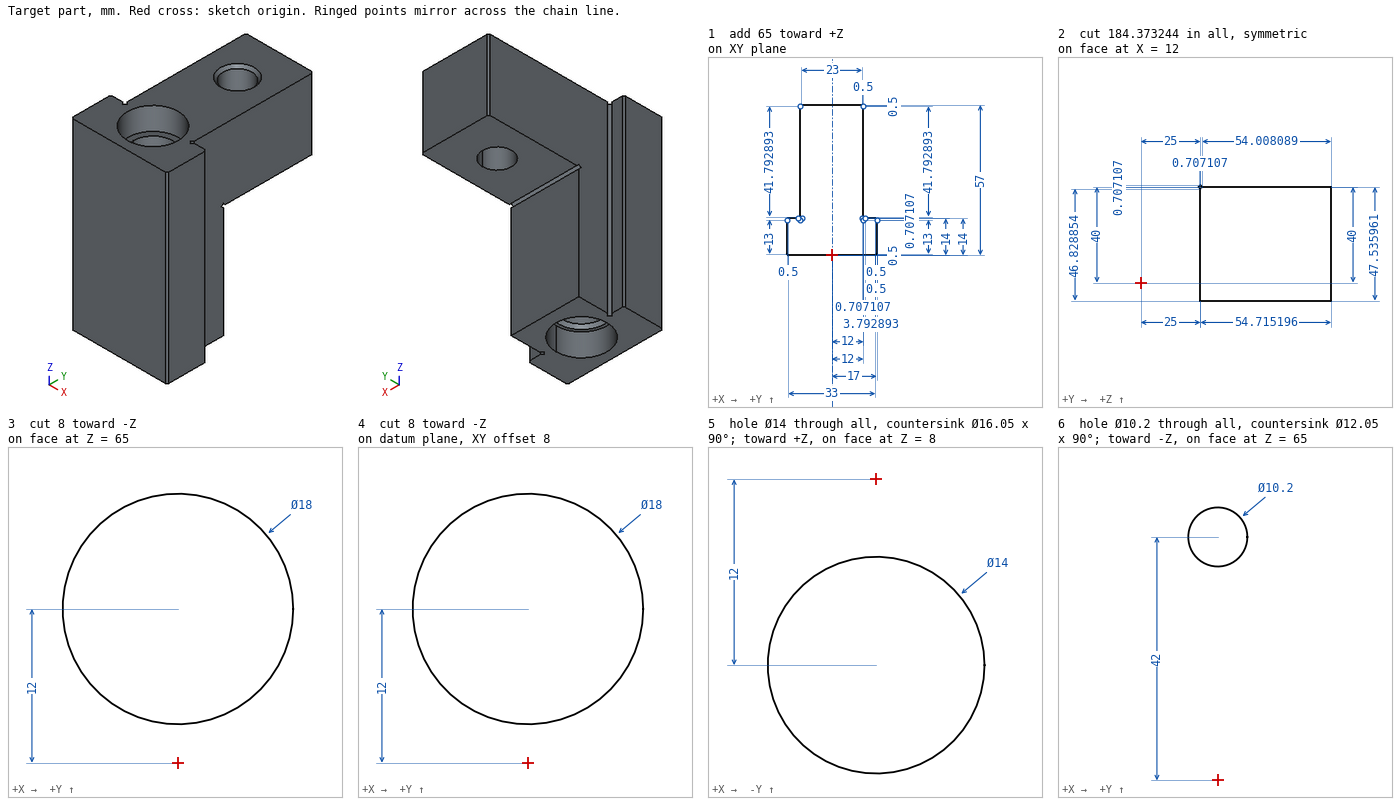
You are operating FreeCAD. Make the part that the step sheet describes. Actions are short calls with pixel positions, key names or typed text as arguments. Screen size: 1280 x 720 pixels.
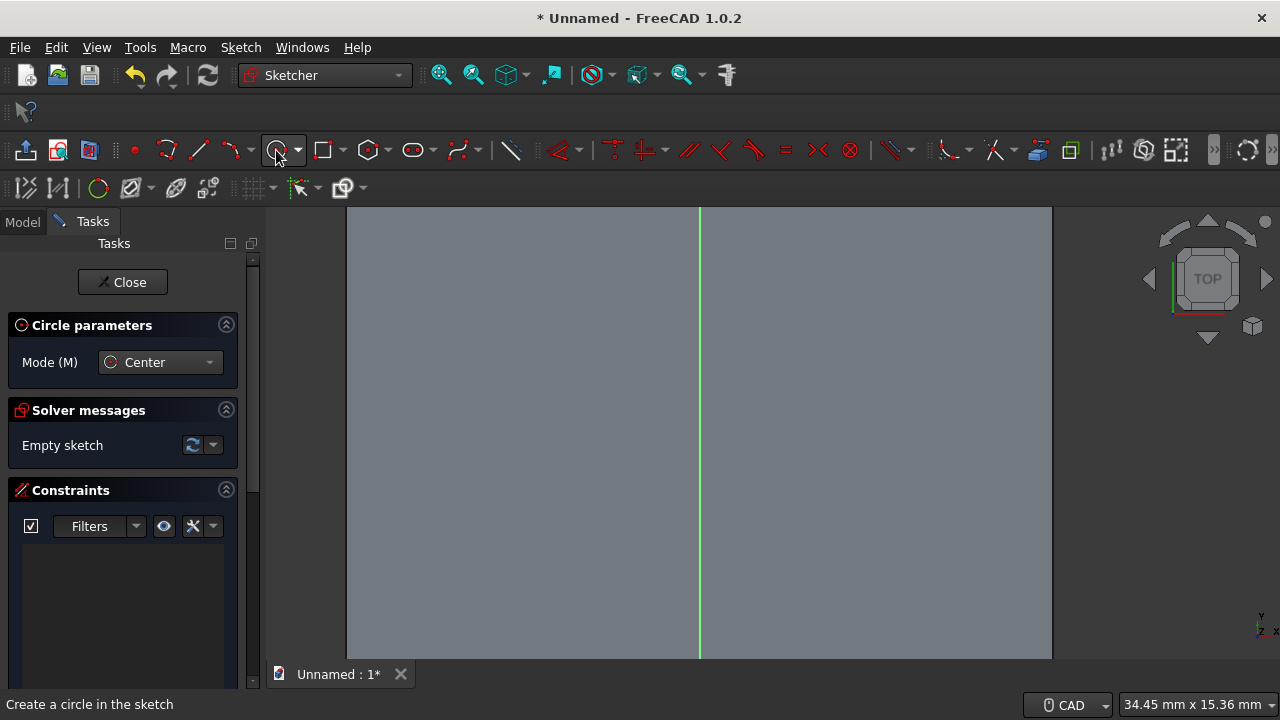
click(700, 433)
click(806, 327)
key(Escape)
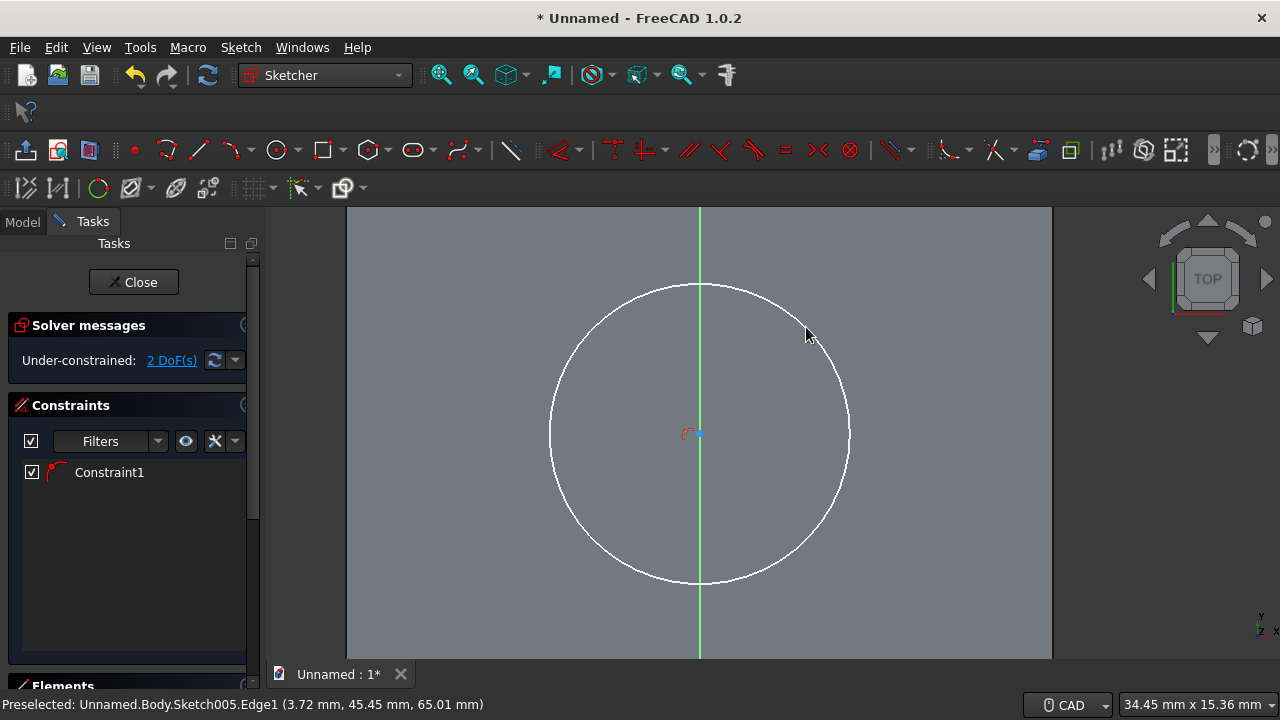
key(d)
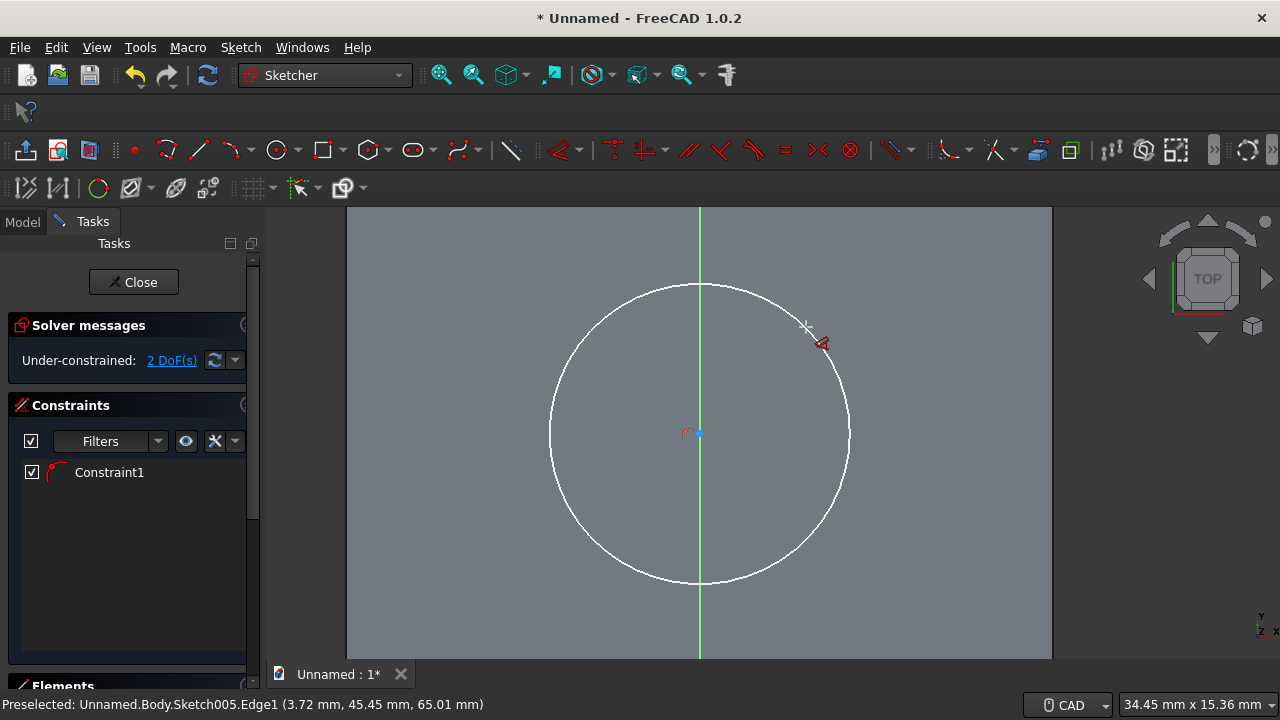
click(806, 328)
click(829, 305)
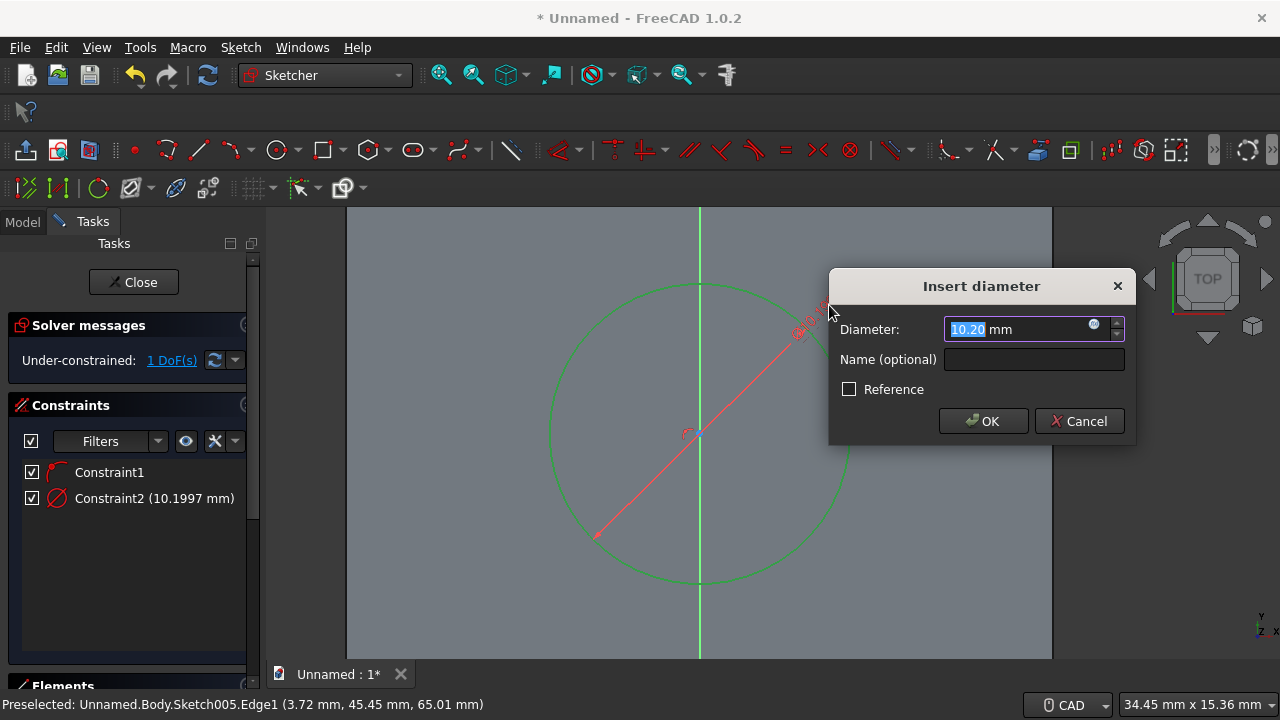
text(10.2)
key(Return)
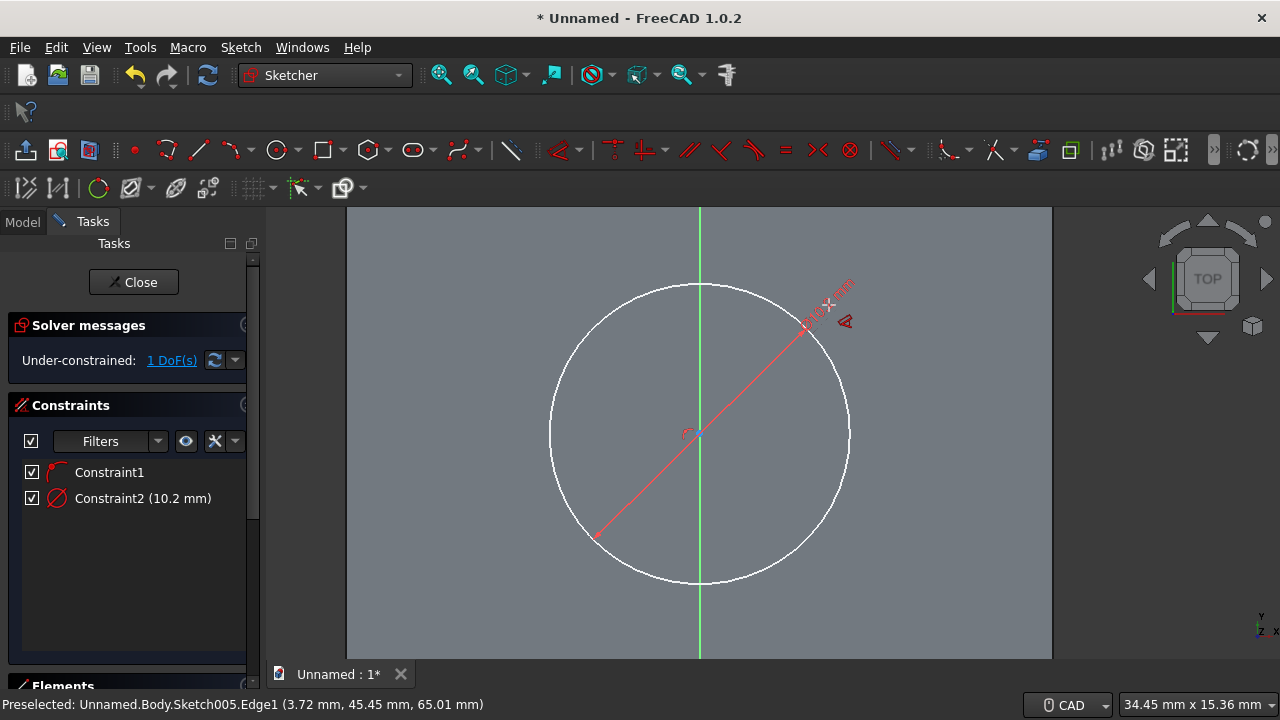
click(700, 434)
click(734, 533)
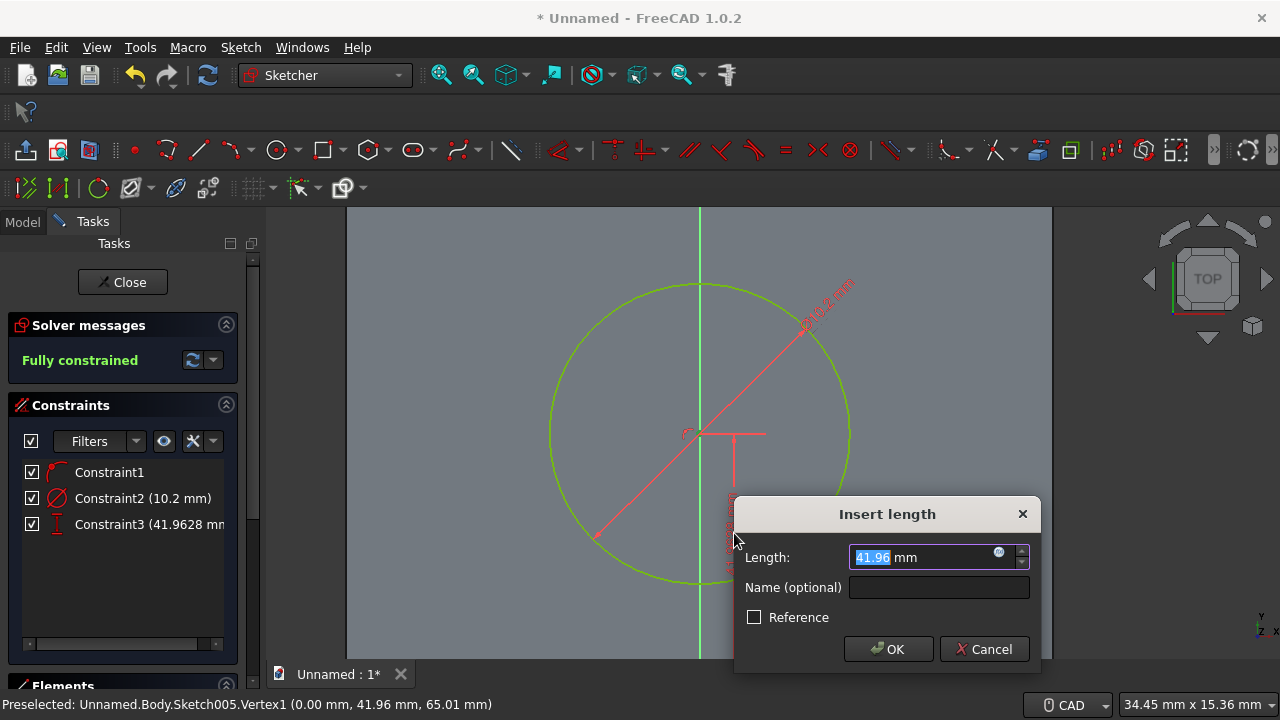
text(42)
key(Return)
key(Escape)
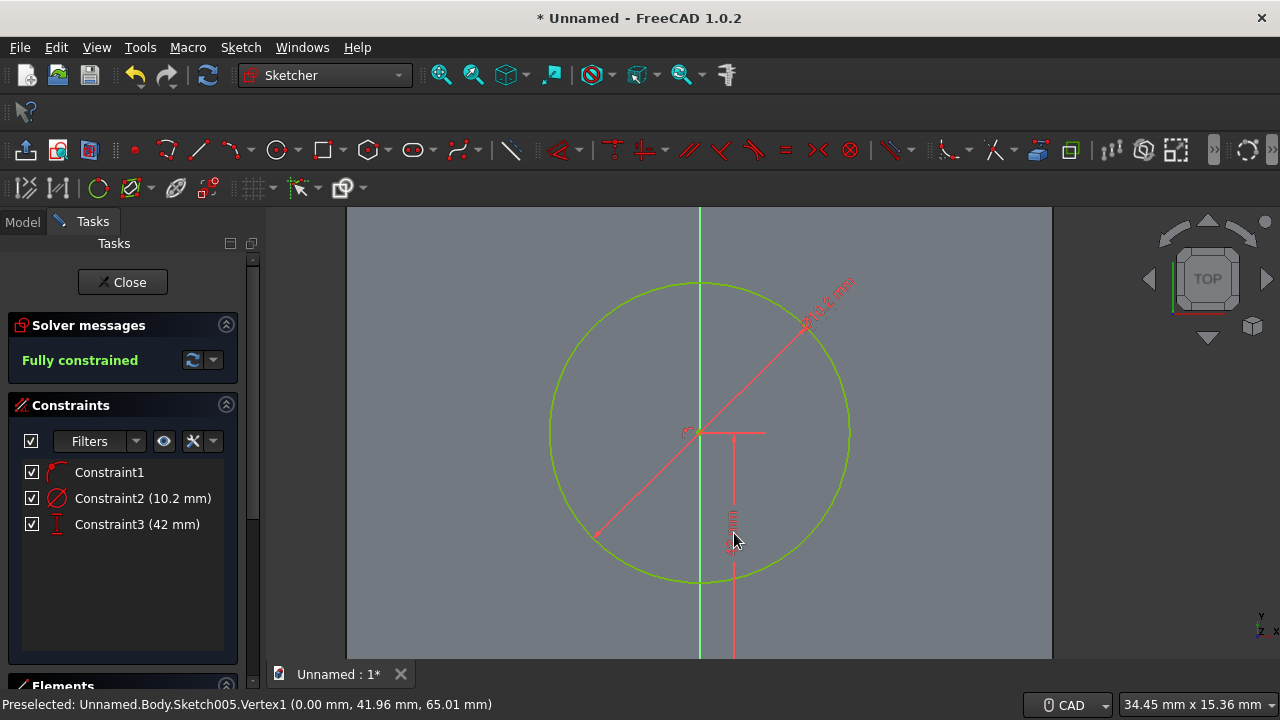
click(123, 282)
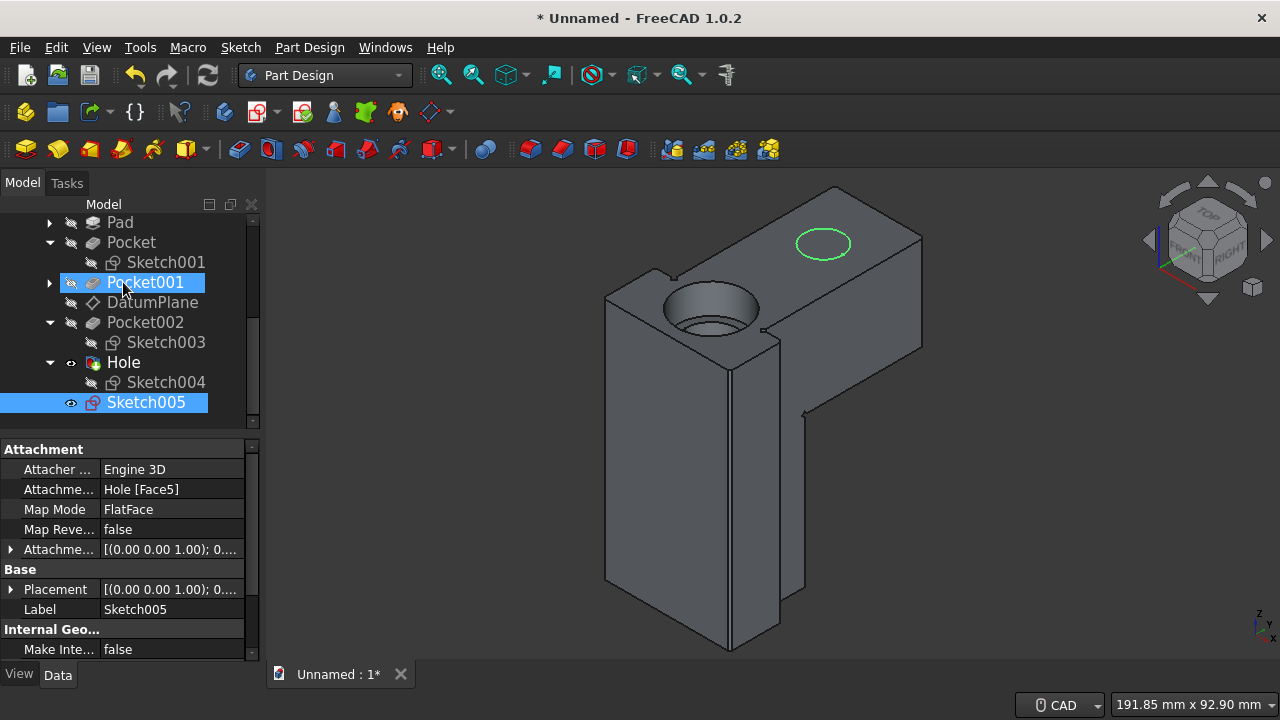
click(272, 150)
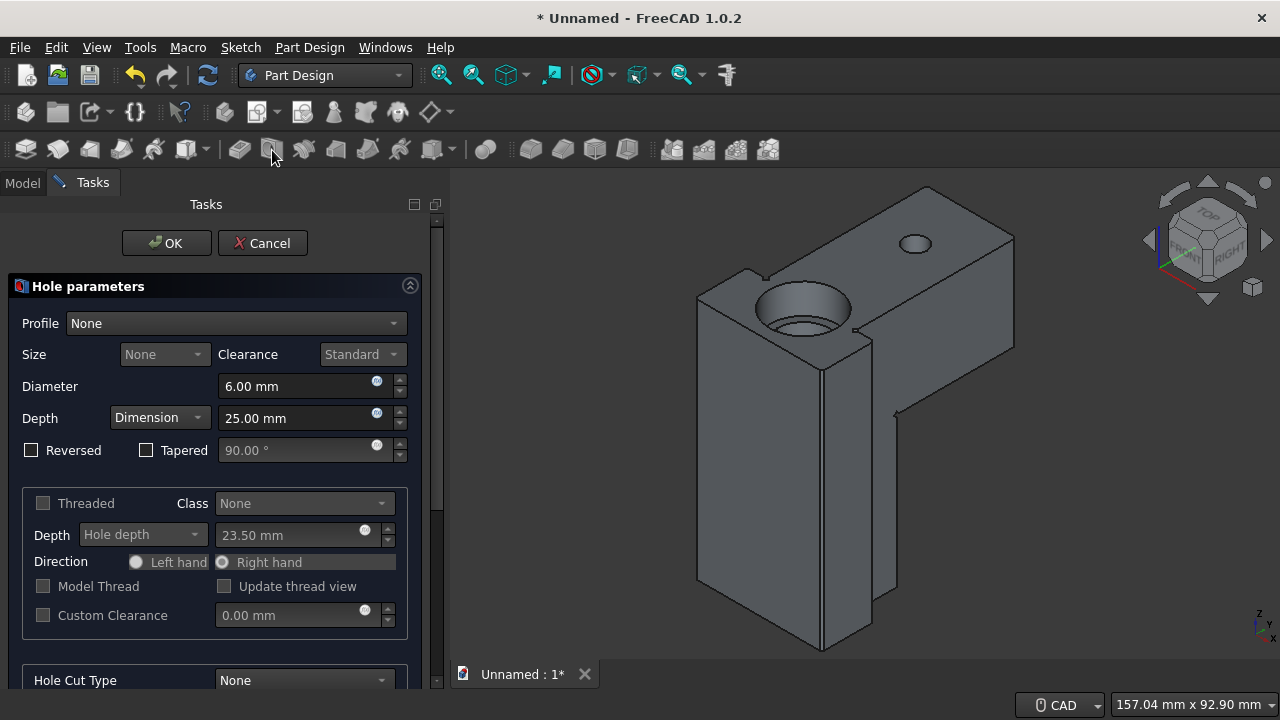
triple_click(305, 386)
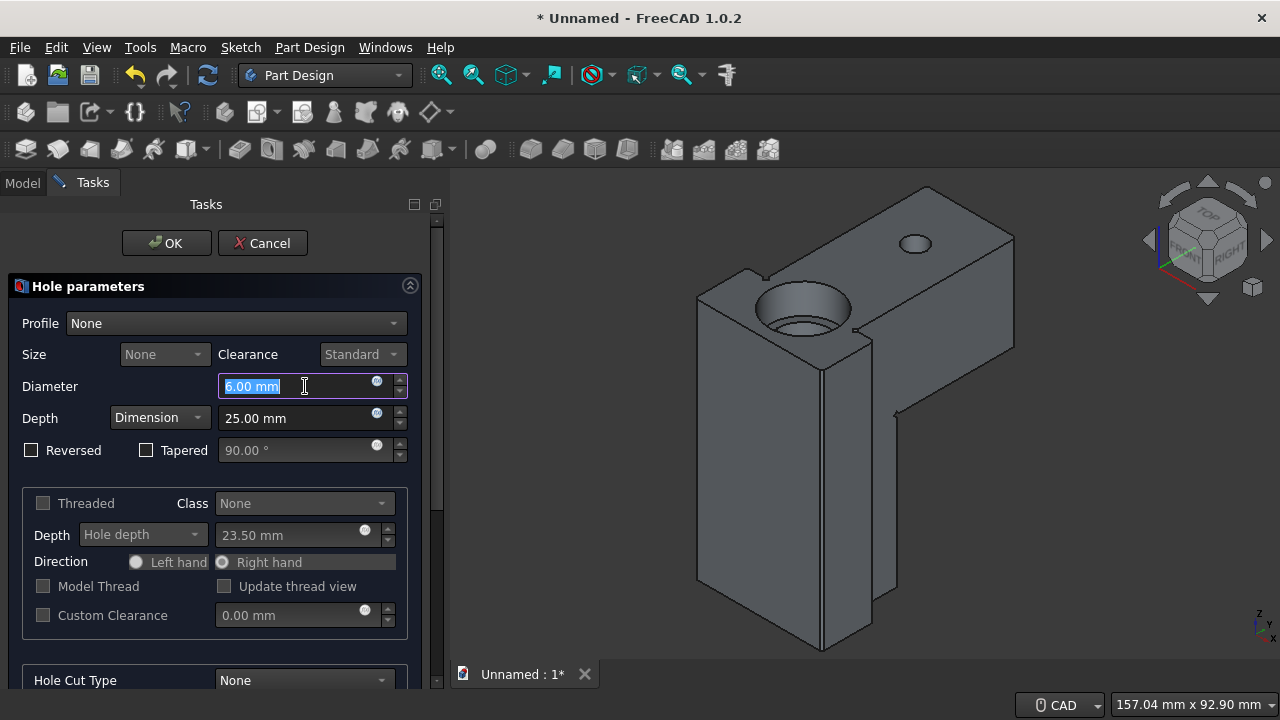
text(10.2)
key(Tab)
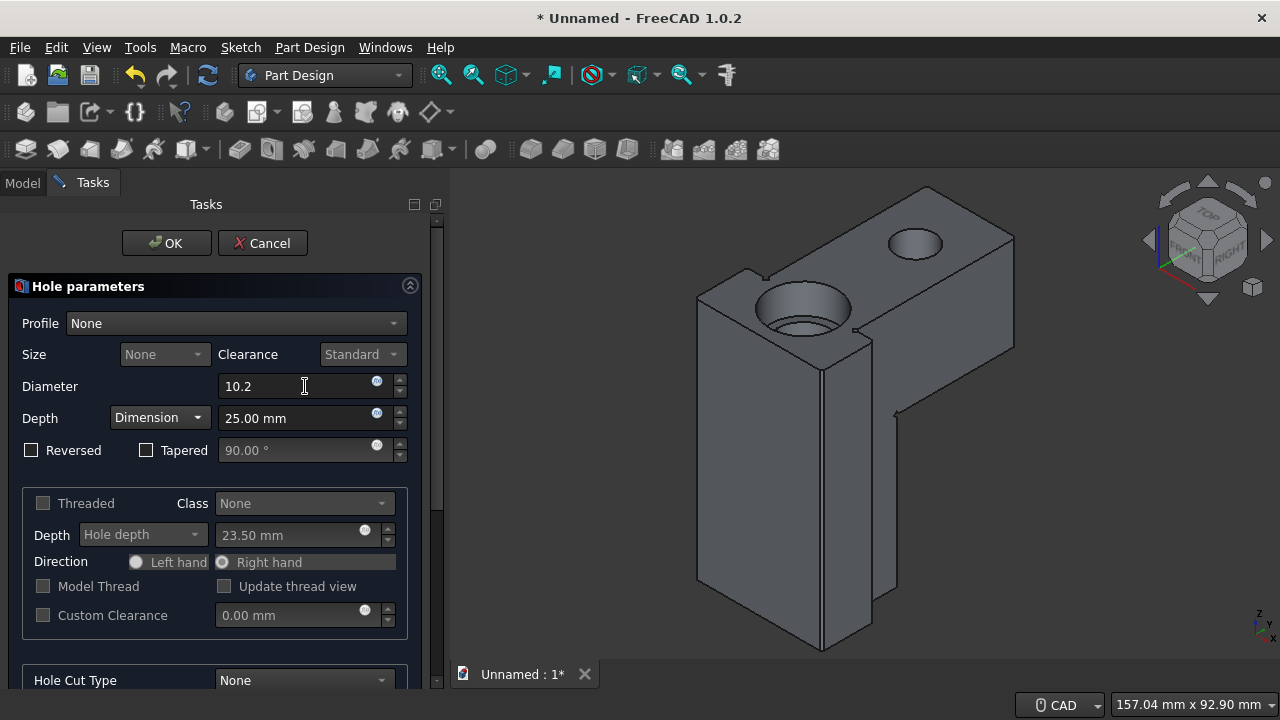
click(161, 418)